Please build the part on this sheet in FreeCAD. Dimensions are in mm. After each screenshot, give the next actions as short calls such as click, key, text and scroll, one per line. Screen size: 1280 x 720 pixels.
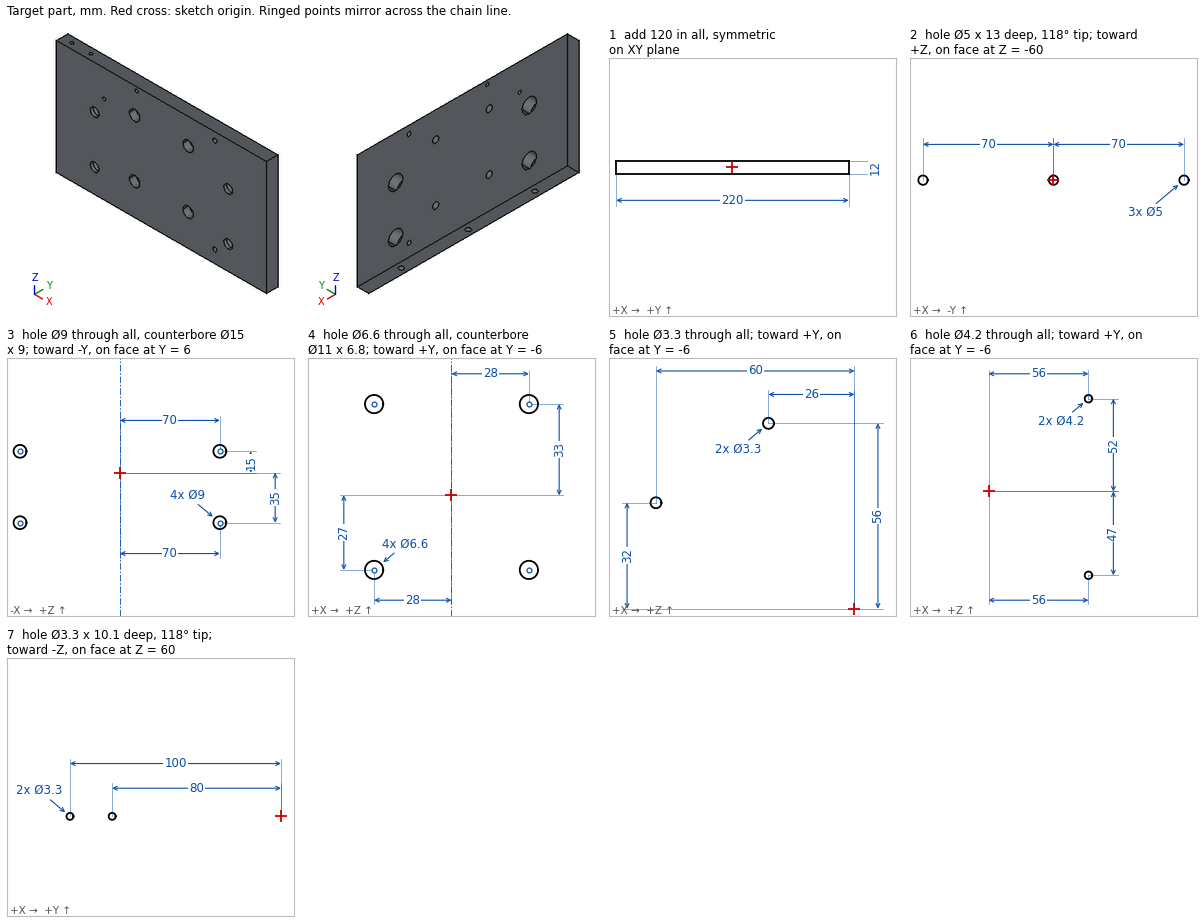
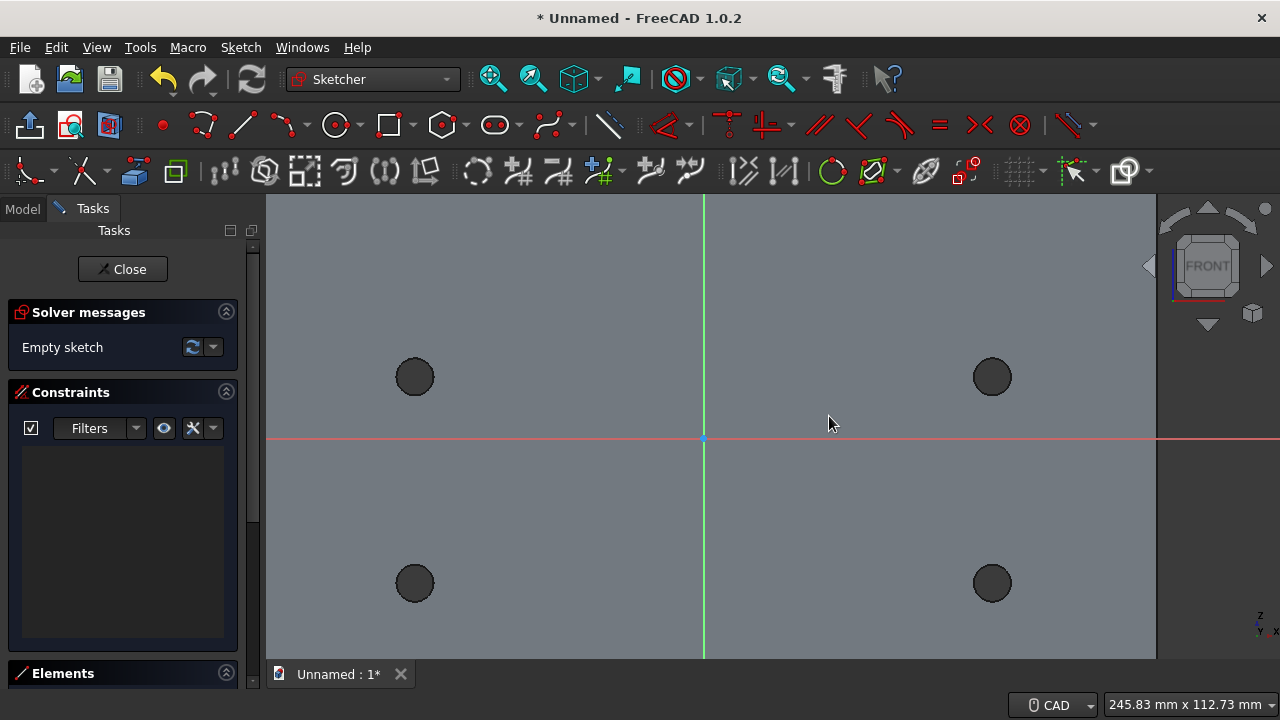
click(336, 126)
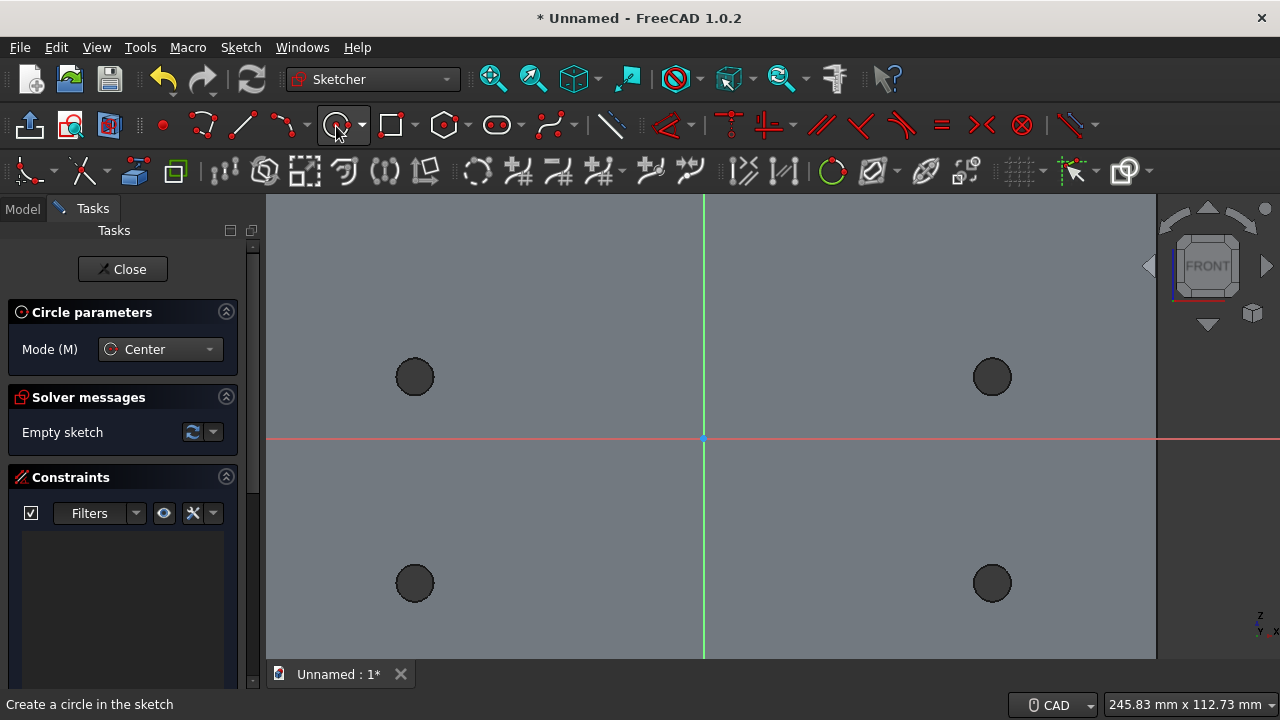
scroll(588, 550, up, 3)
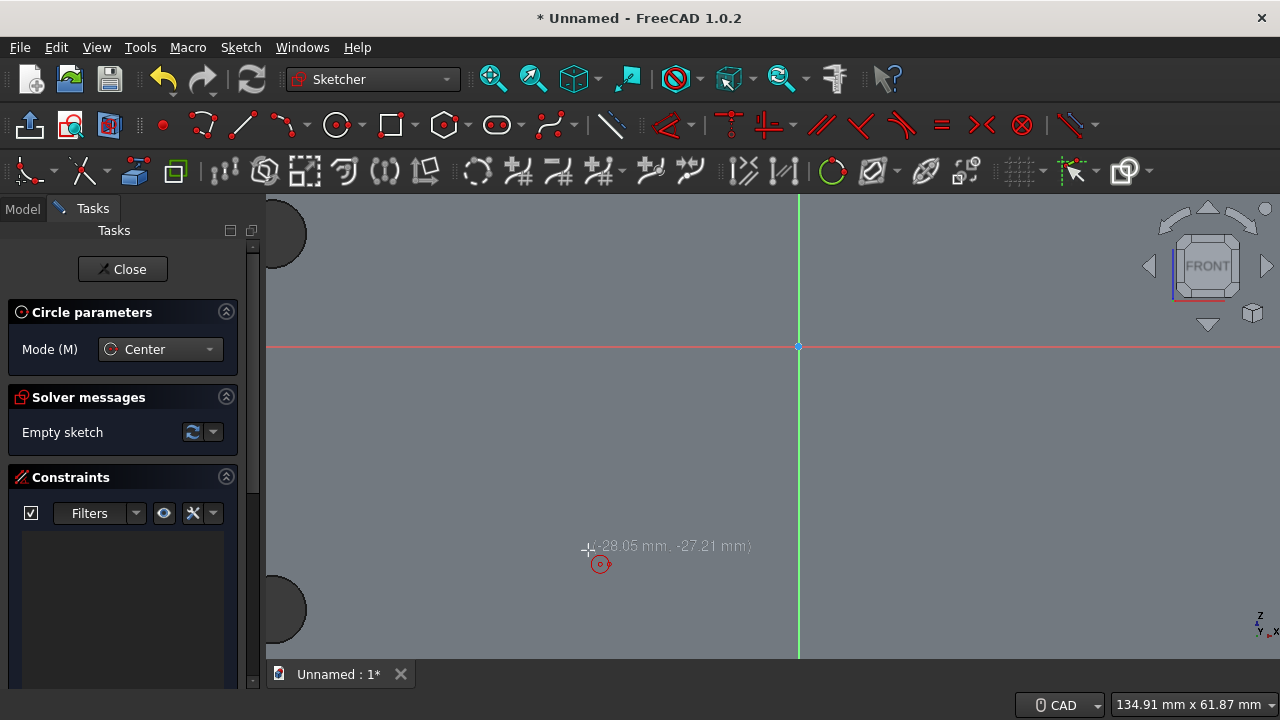
click(588, 550)
move(606, 532)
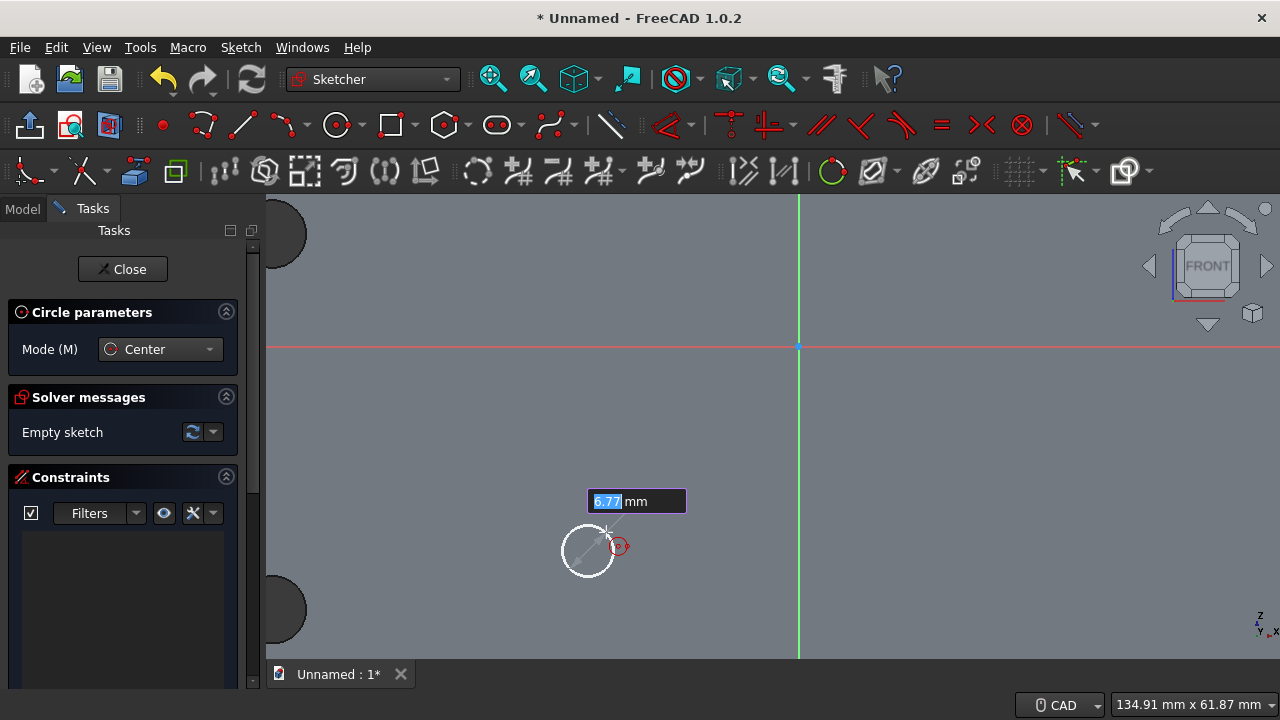
text(6.6)
key(Return)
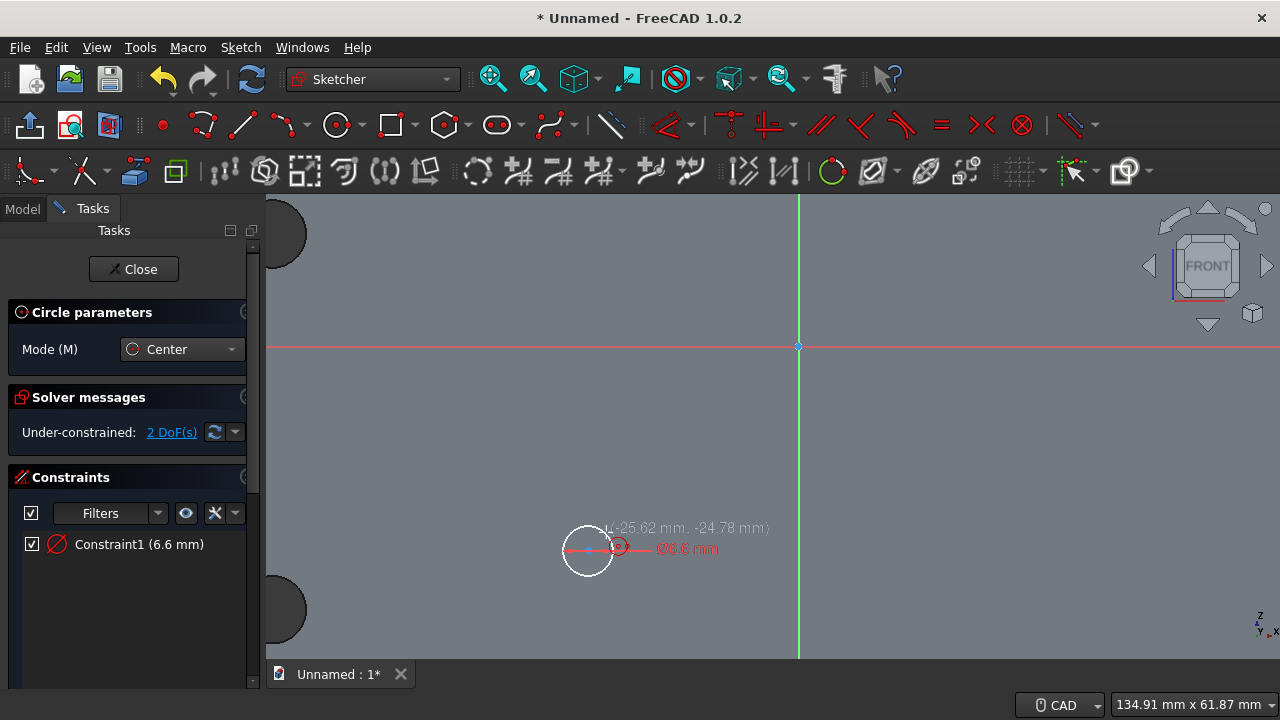
click(1009, 550)
move(1027, 532)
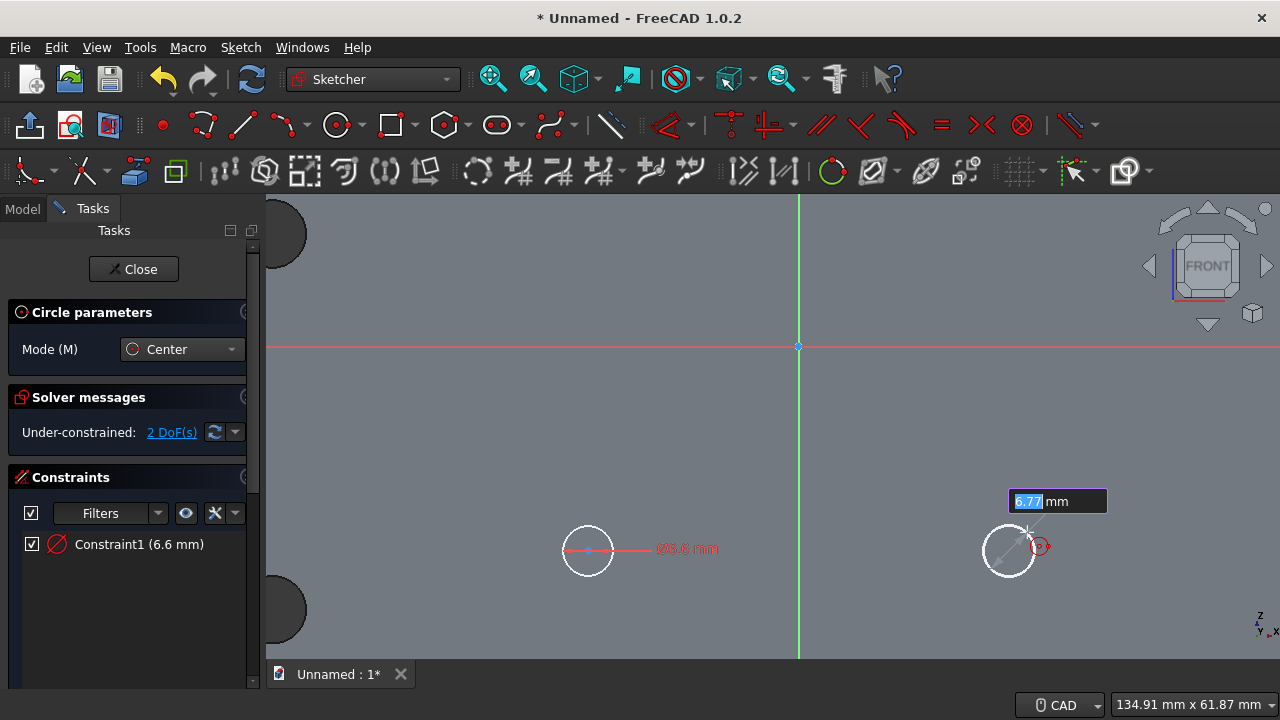
text(6.6)
key(Return)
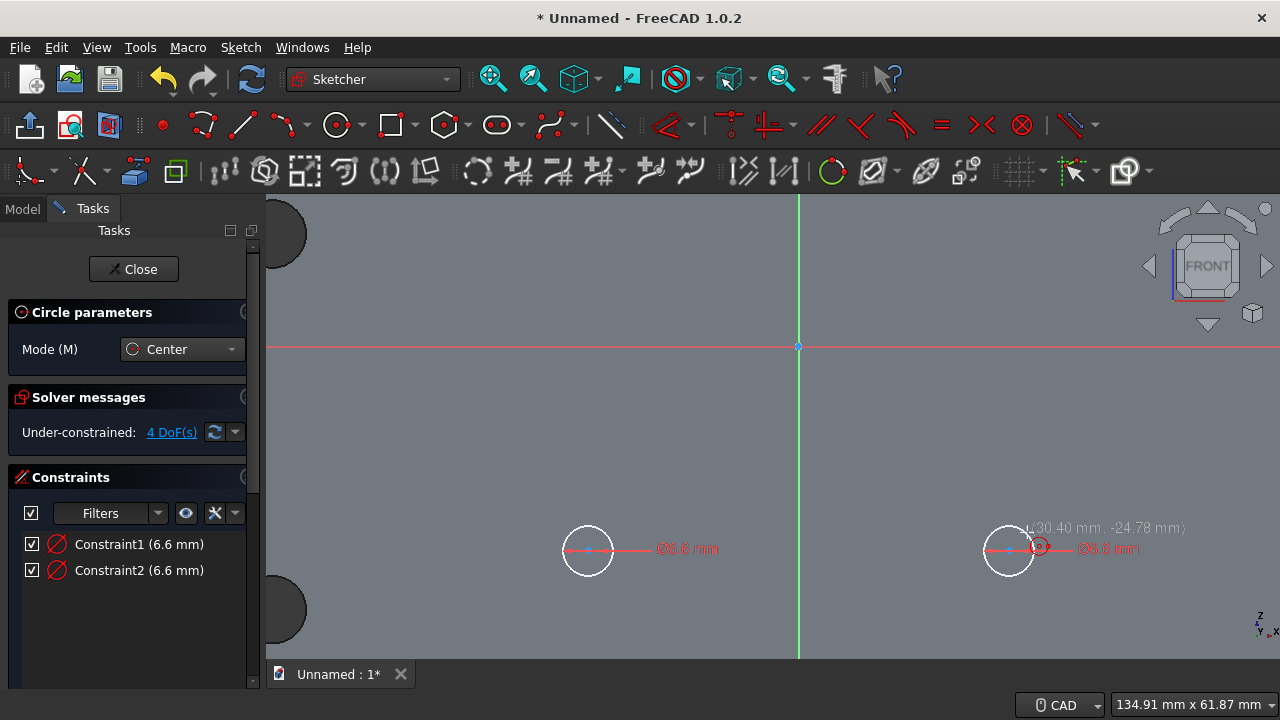
scroll(590, 551, down, 3)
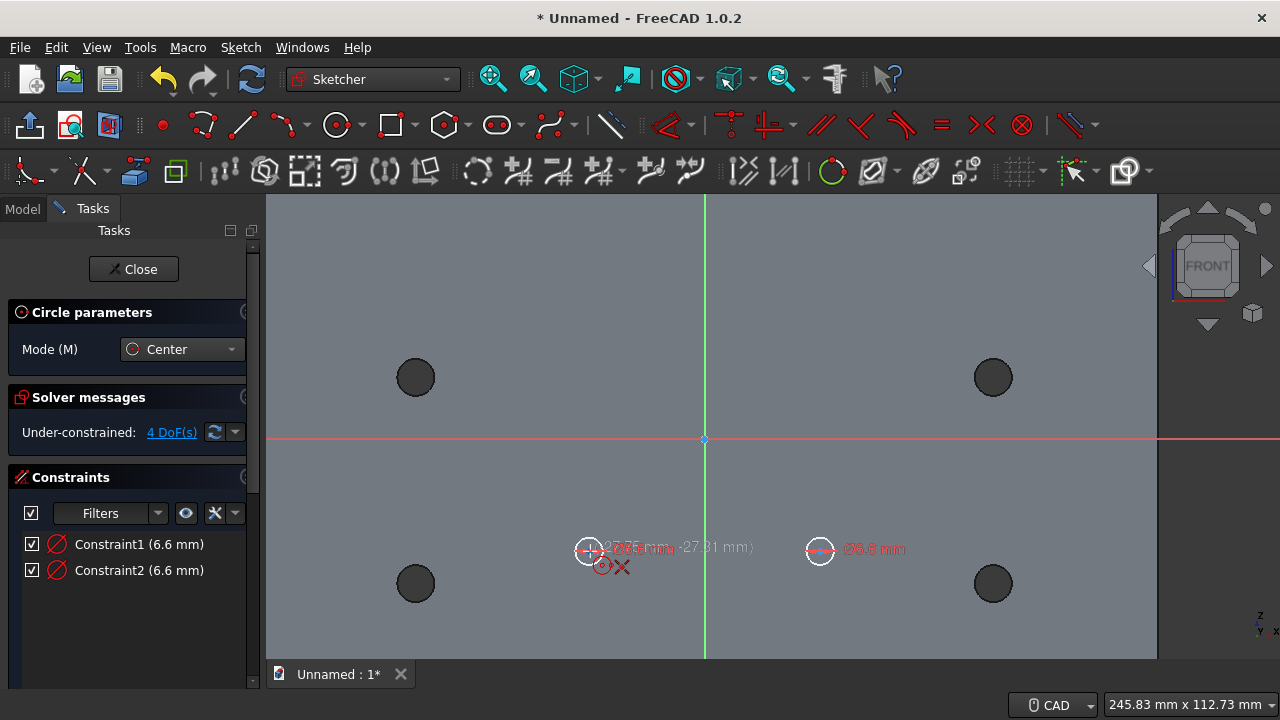
scroll(820, 303, up, 3)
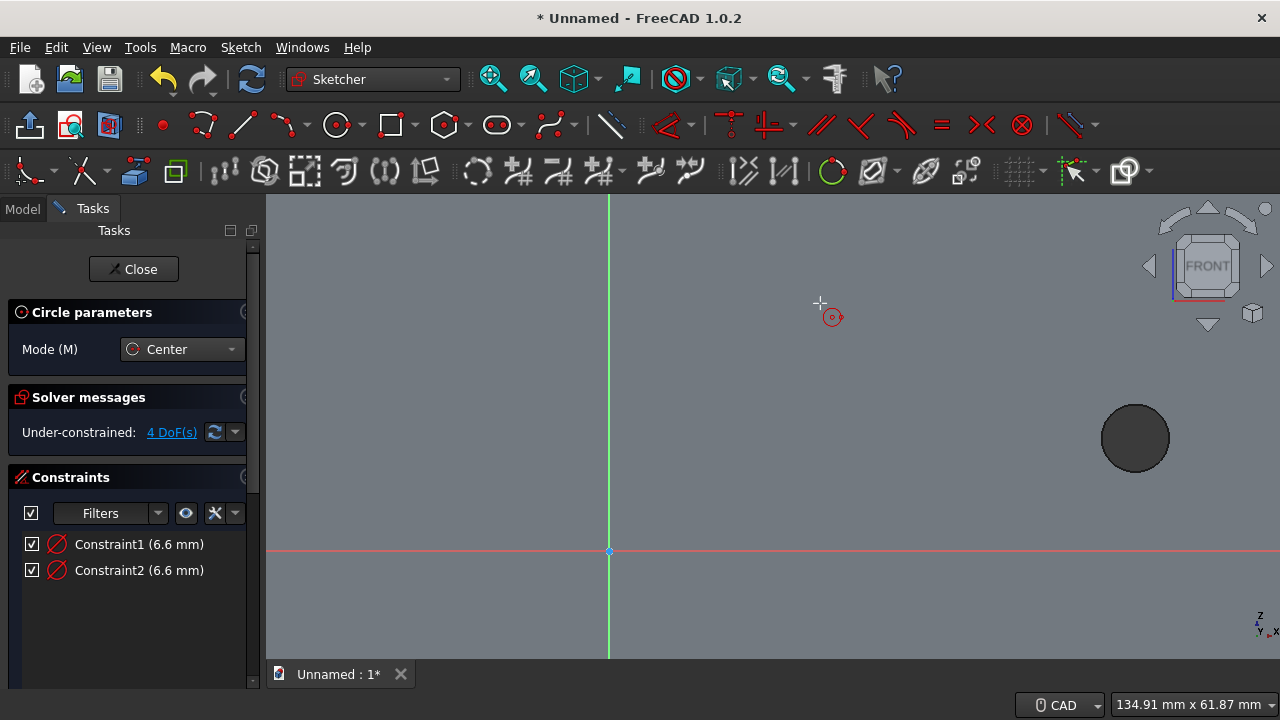
click(820, 303)
move(837, 285)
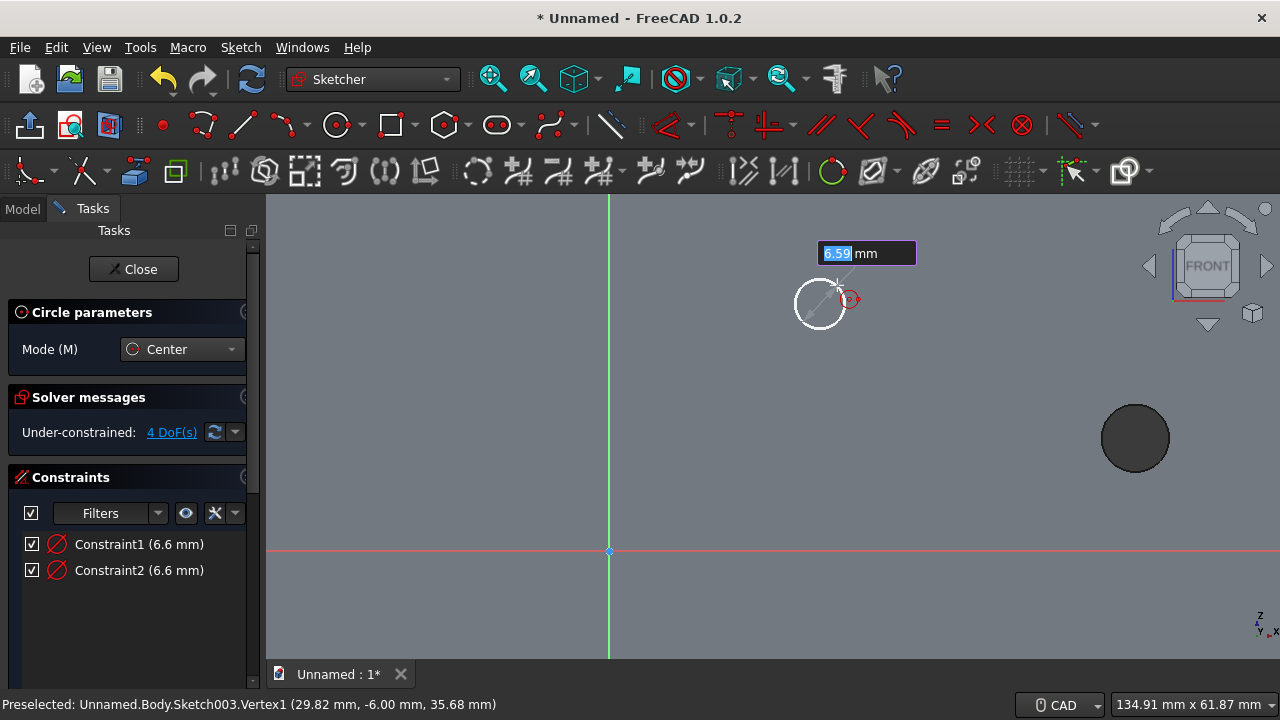
text(6.6)
key(Return)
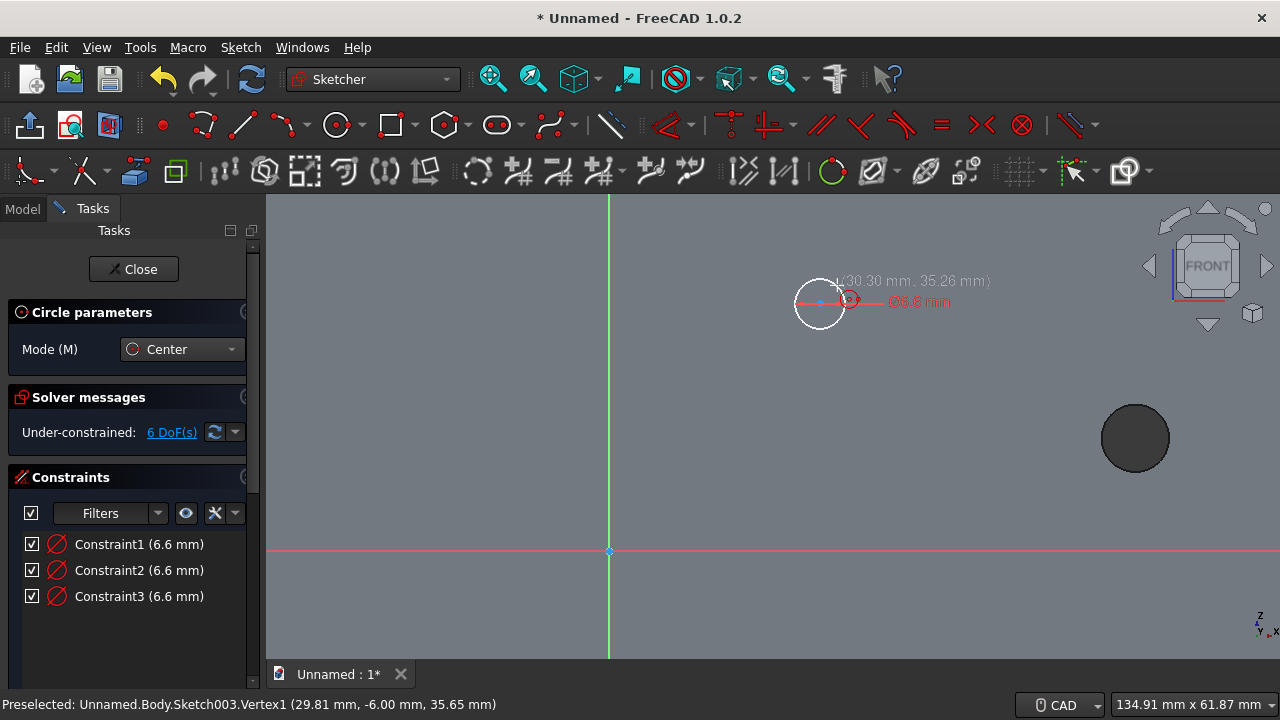
click(399, 303)
move(416, 285)